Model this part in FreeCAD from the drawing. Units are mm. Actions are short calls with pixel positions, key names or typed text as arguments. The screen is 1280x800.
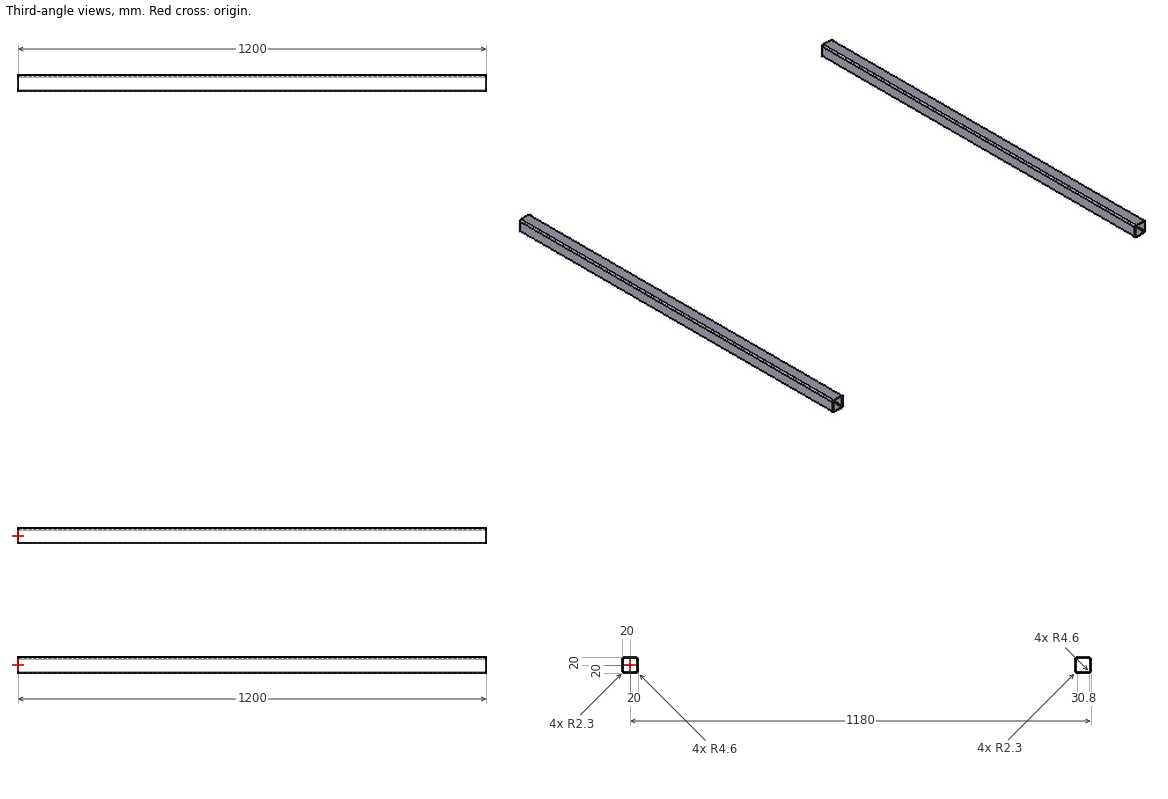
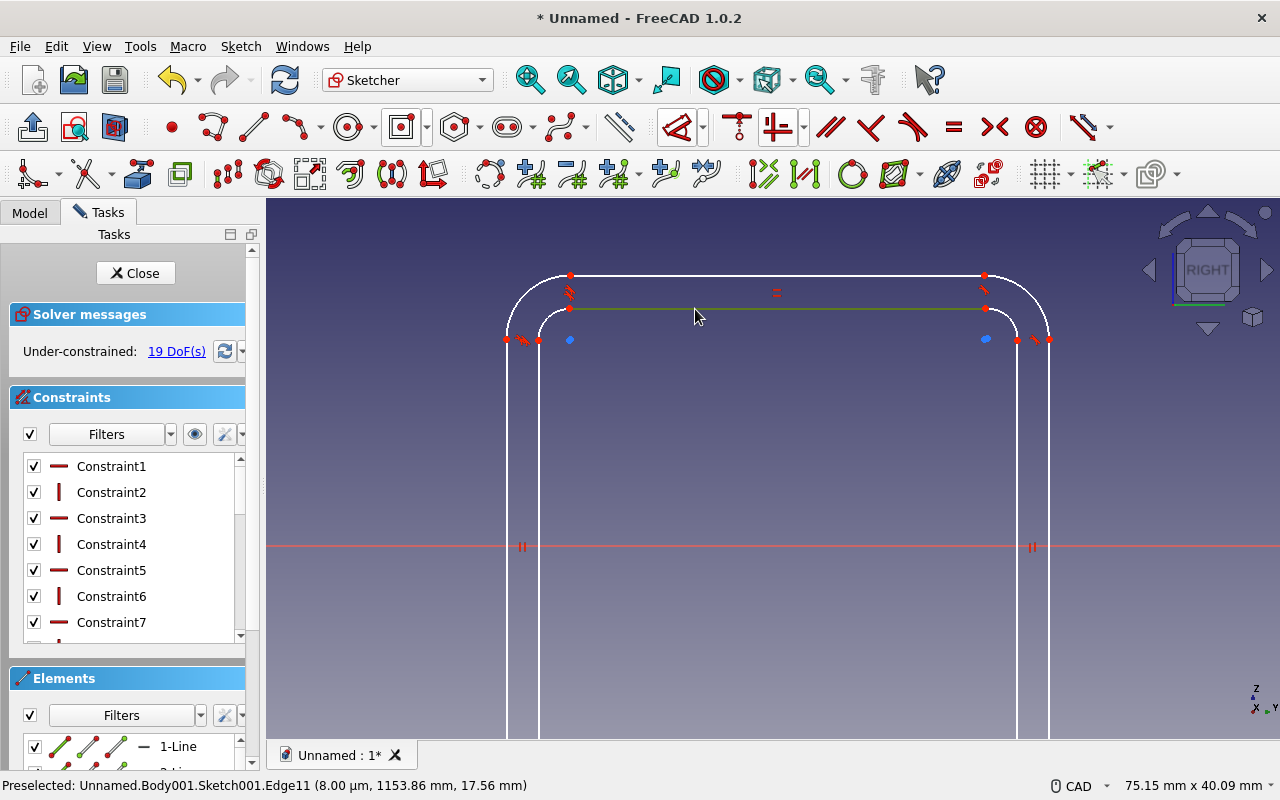
click(1014, 326)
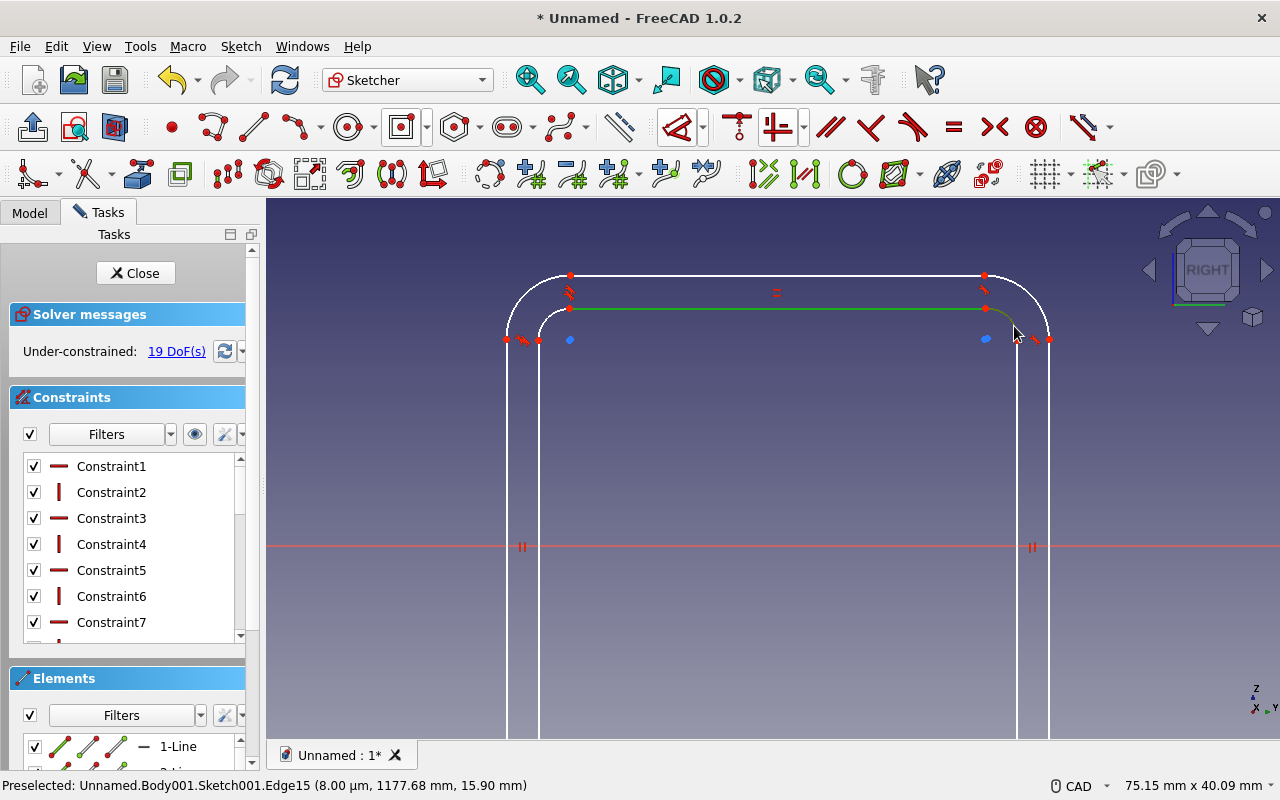
key(t)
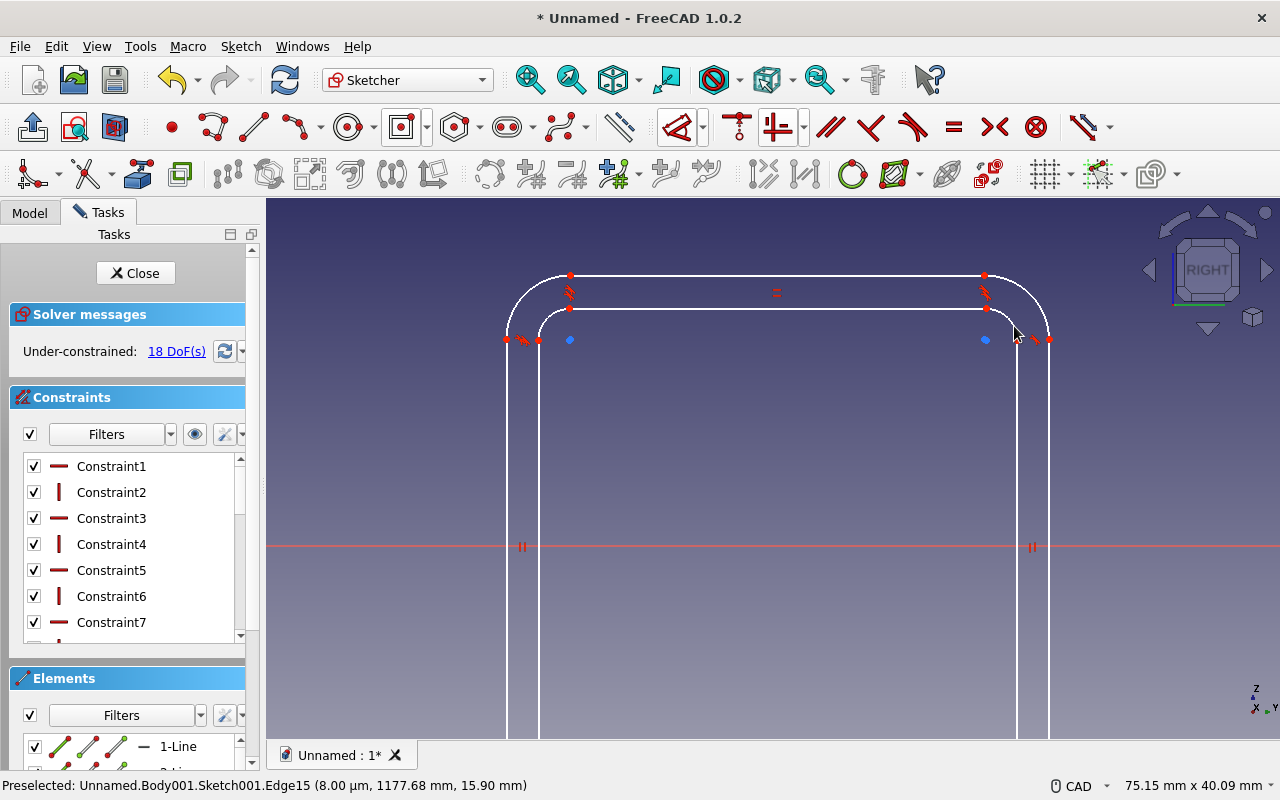
click(1017, 465)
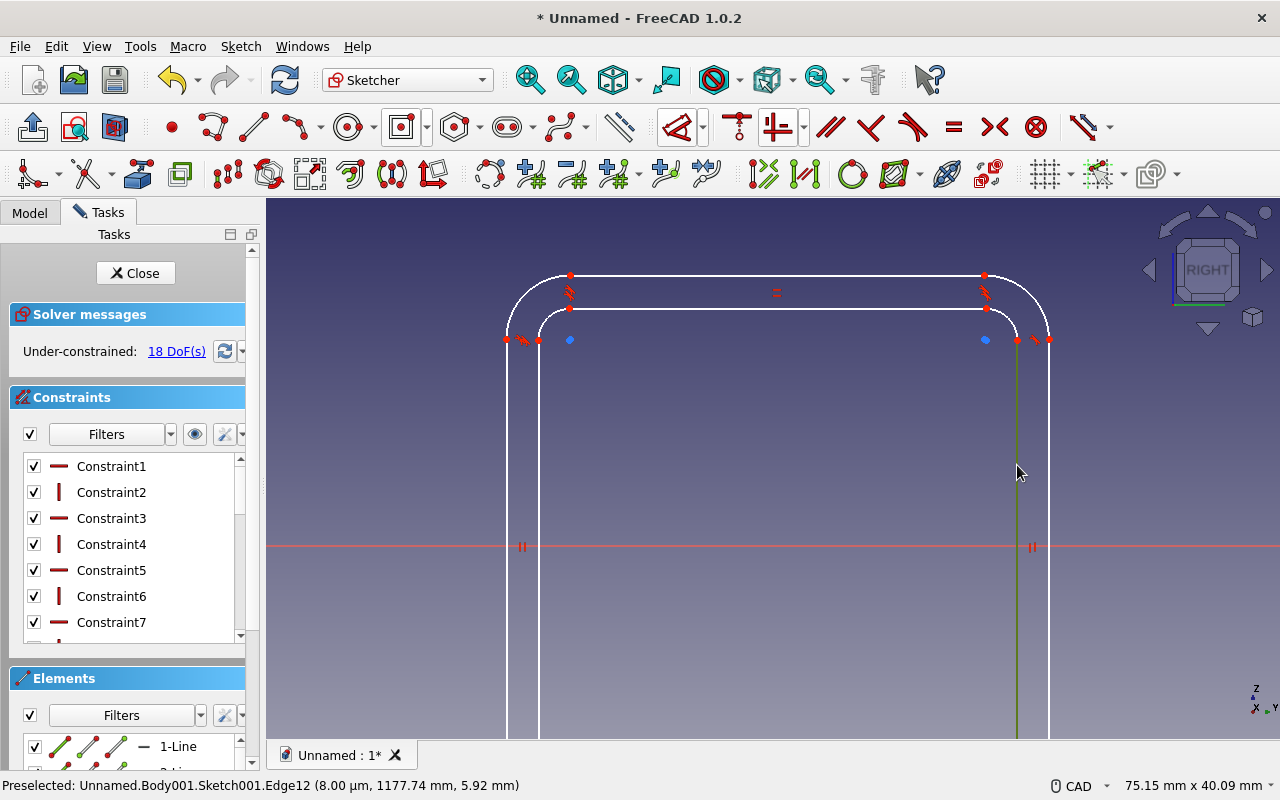
click(1014, 326)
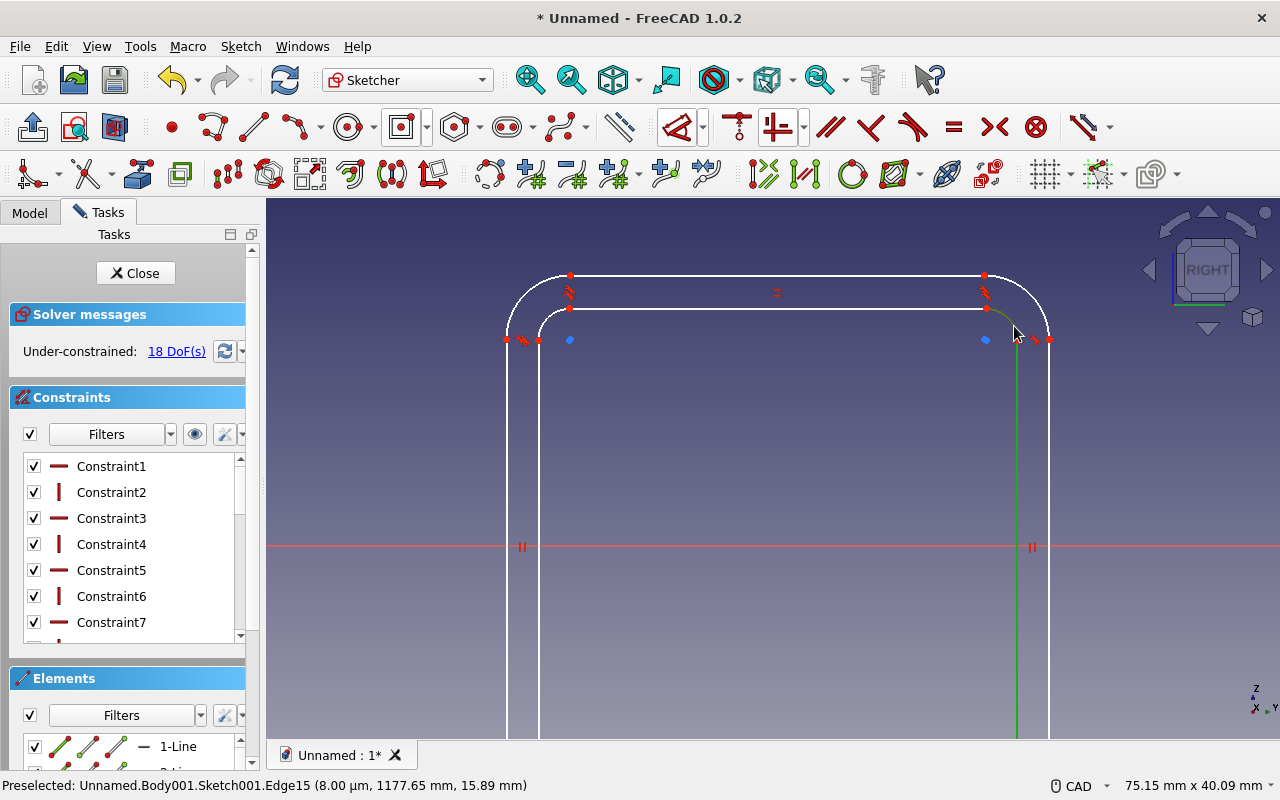
key(t)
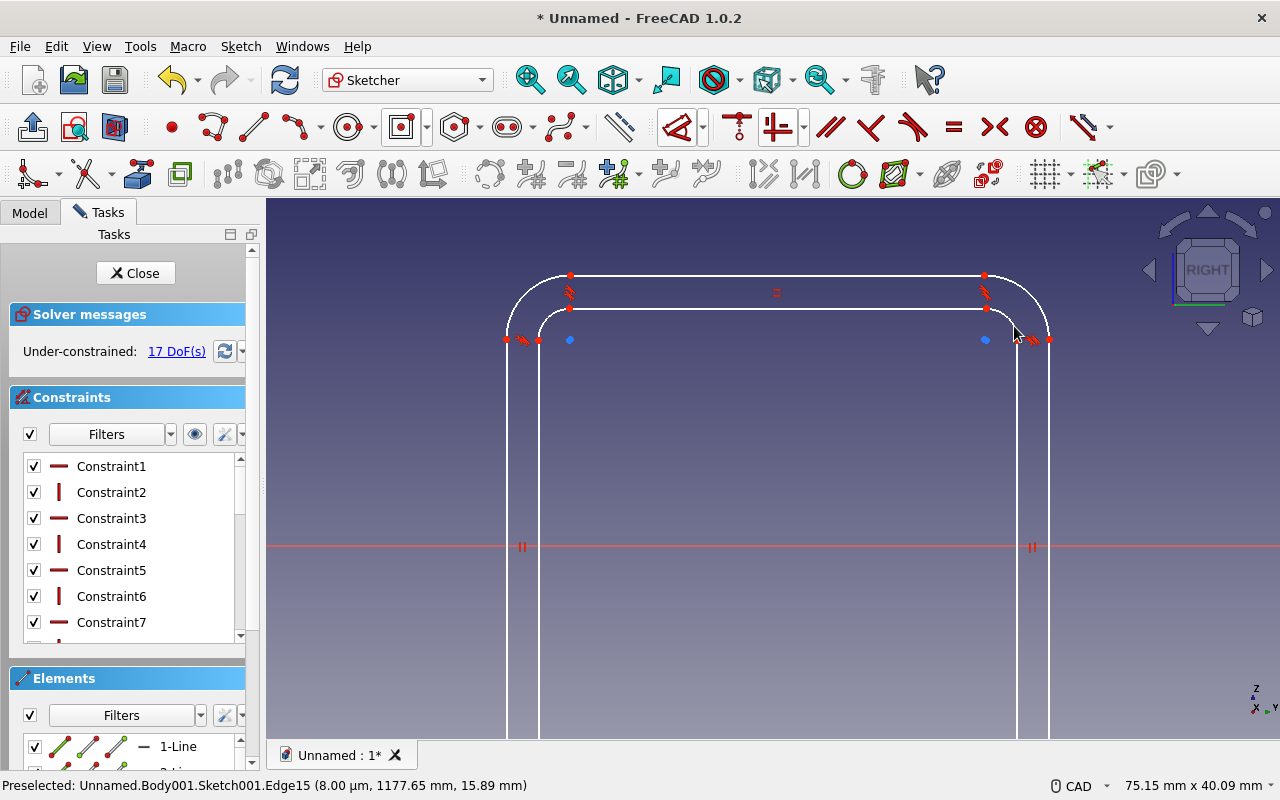
click(1017, 465)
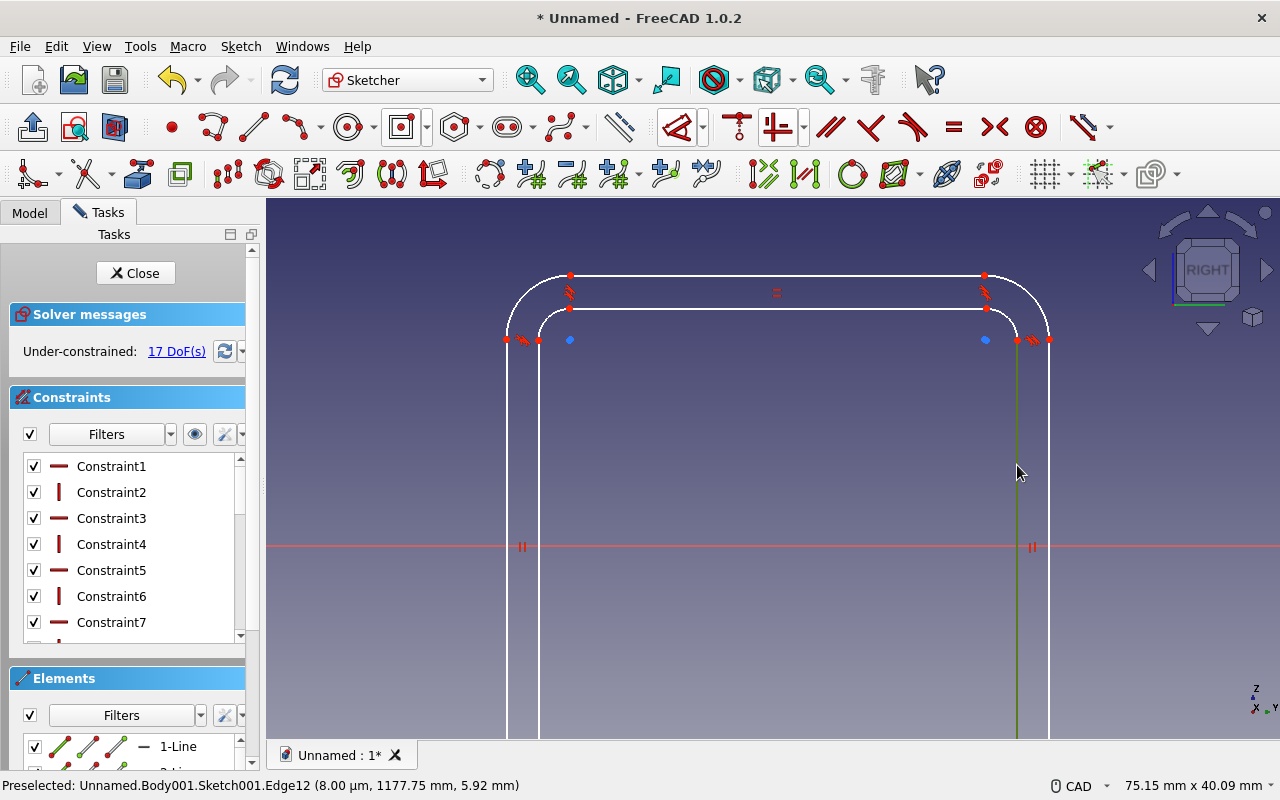
scroll(555, 311, down, 2)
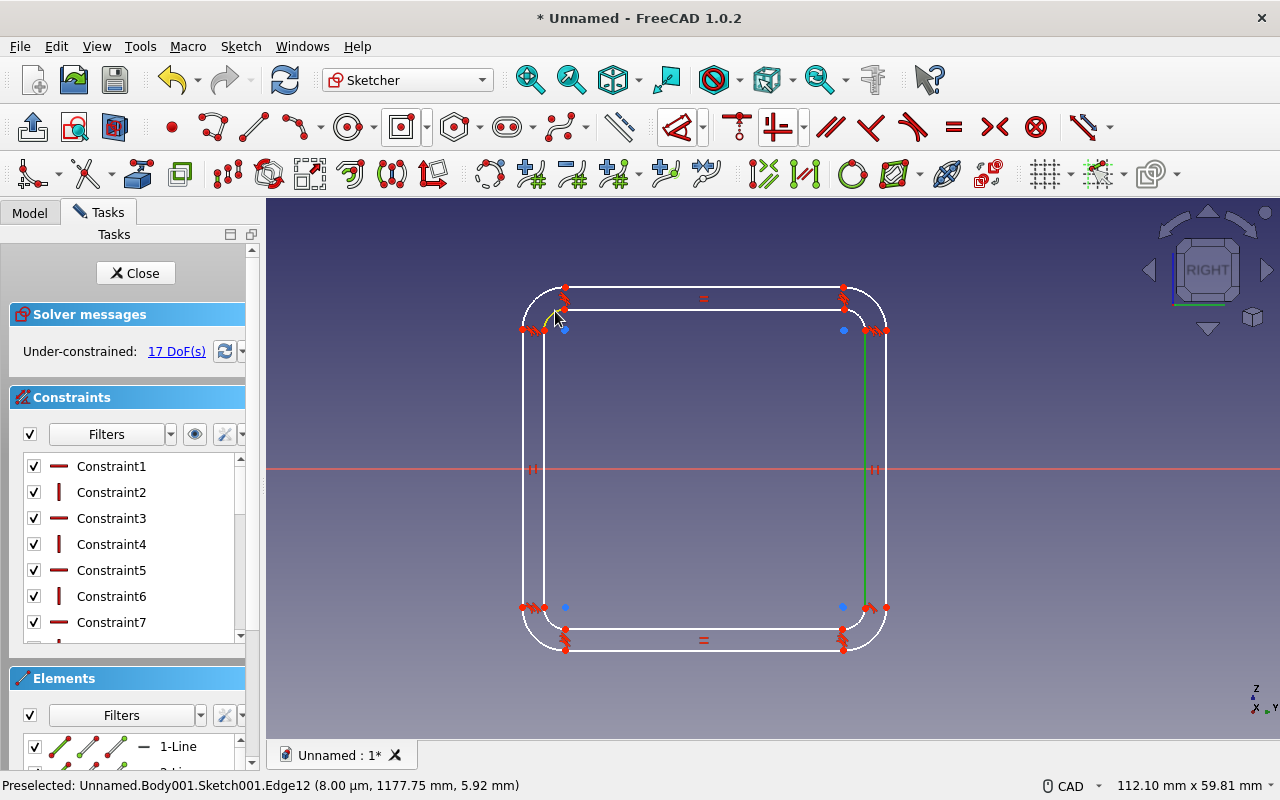
scroll(852, 627, up, 2)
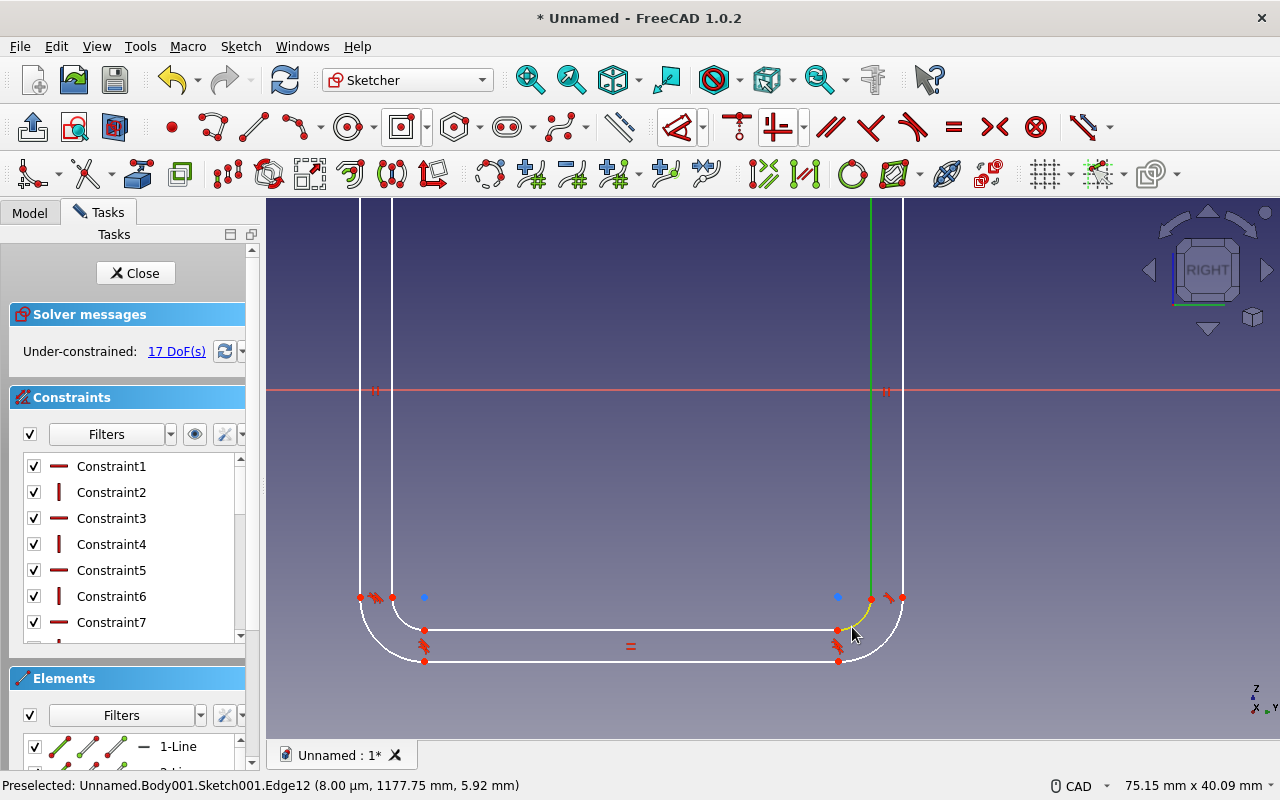
click(852, 627)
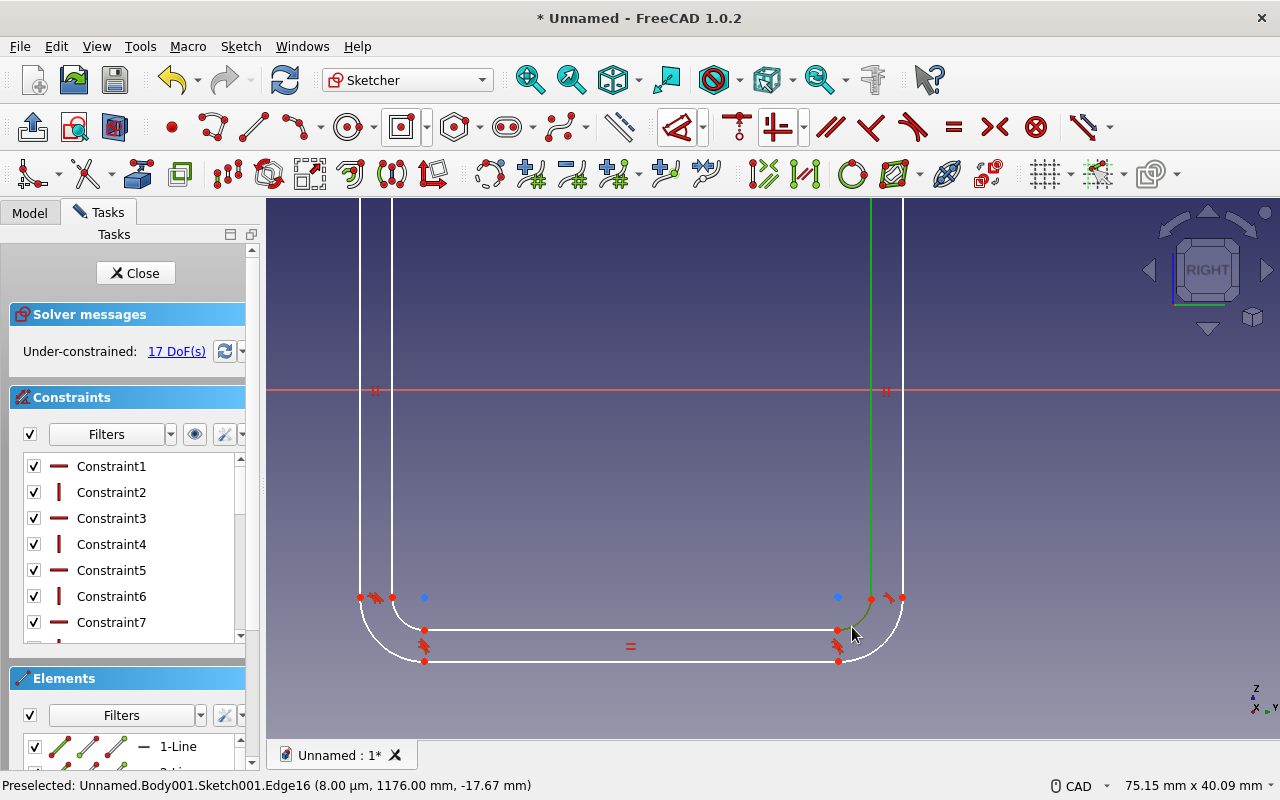
key(t)